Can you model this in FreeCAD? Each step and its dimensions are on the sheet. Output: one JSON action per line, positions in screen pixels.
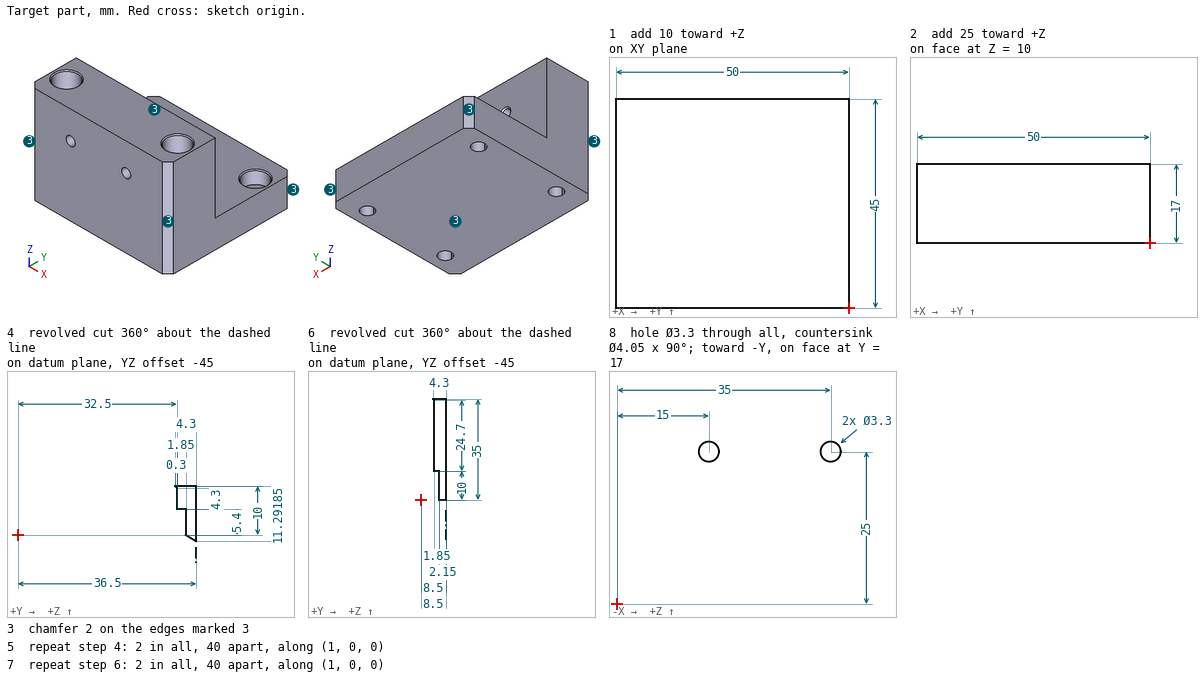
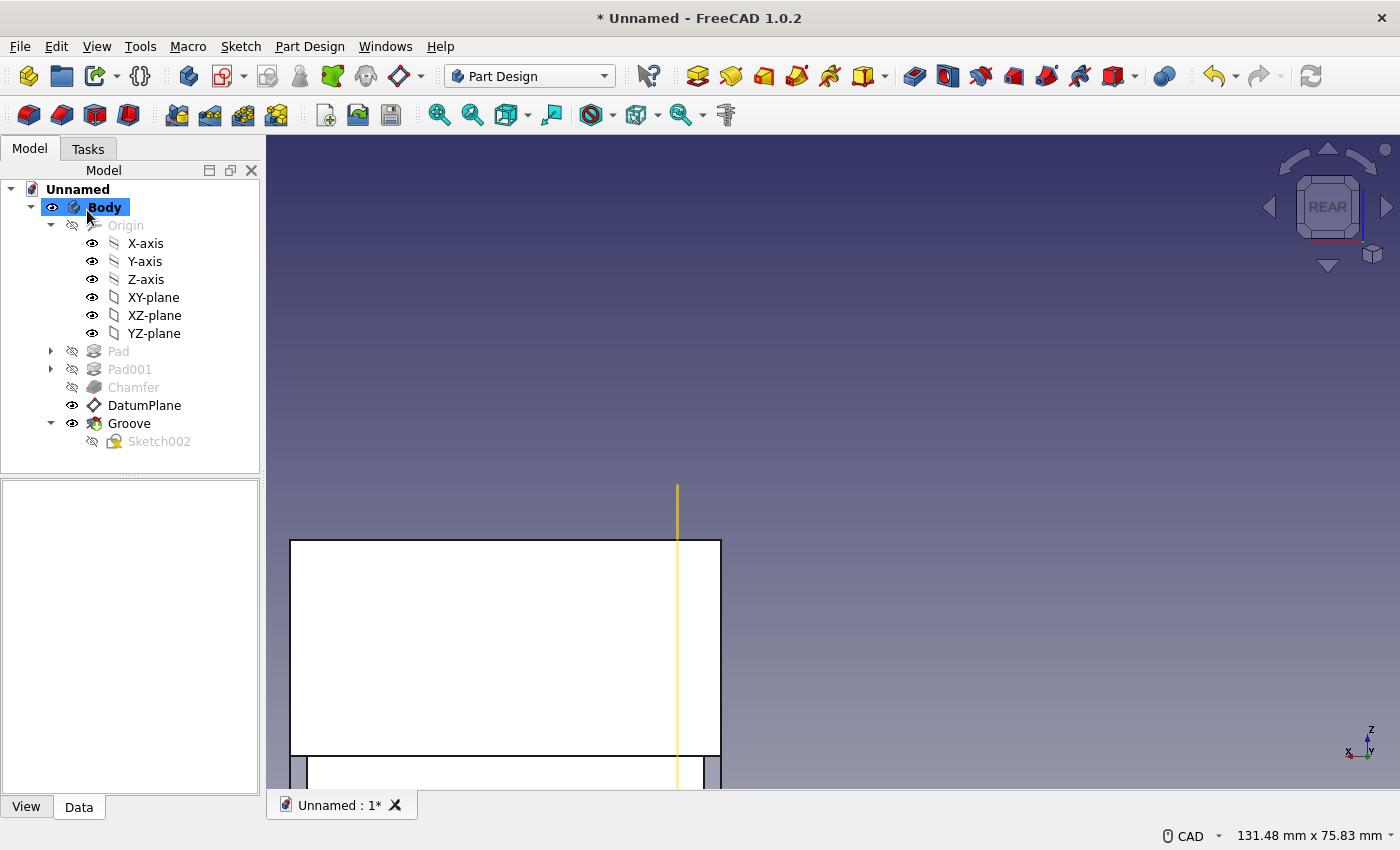
{"action": "left_click", "coordinate": [117, 405]}
{"action": "key", "text": "space"}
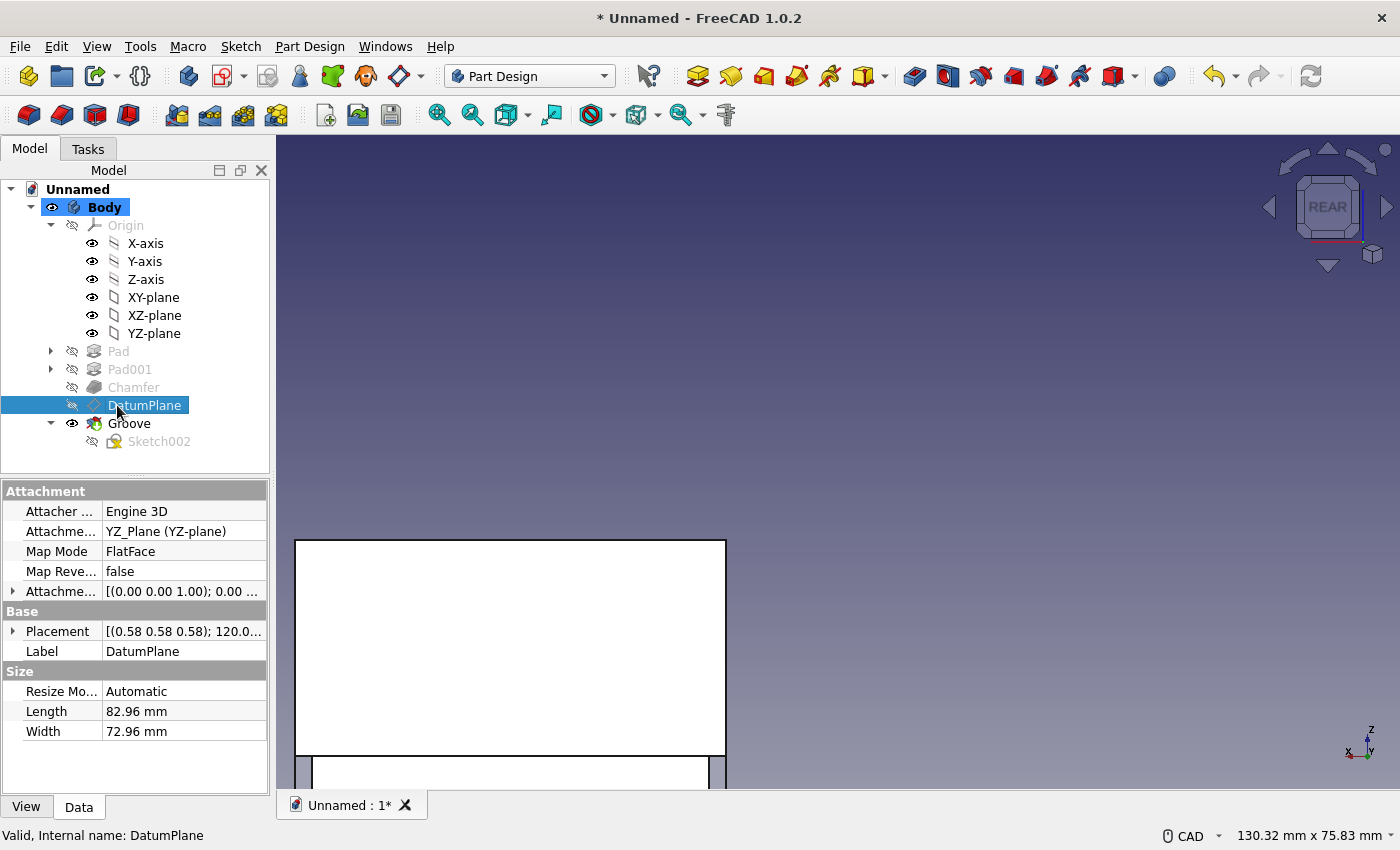
{"action": "key", "text": "v f"}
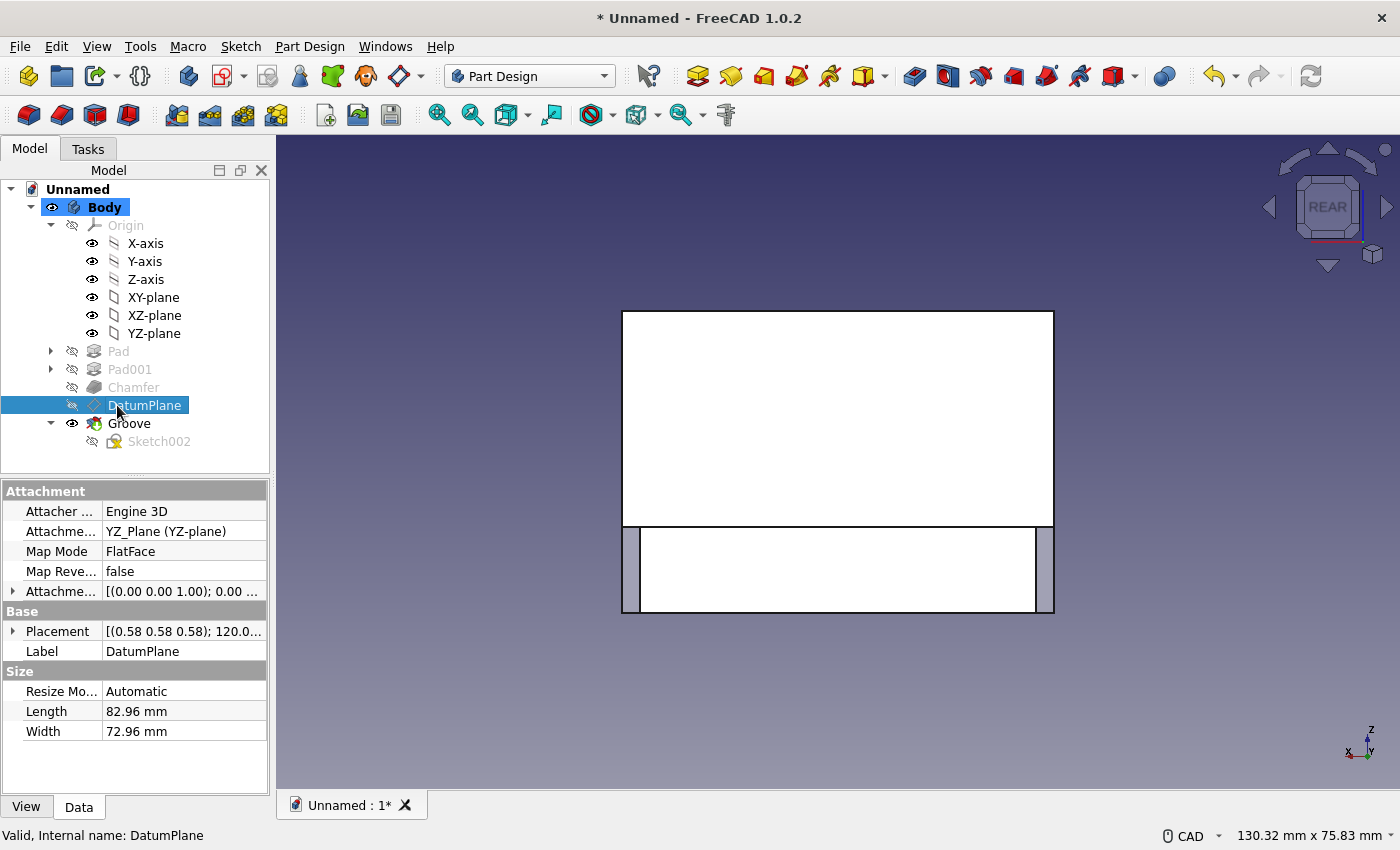
{"action": "left_click", "coordinate": [117, 423]}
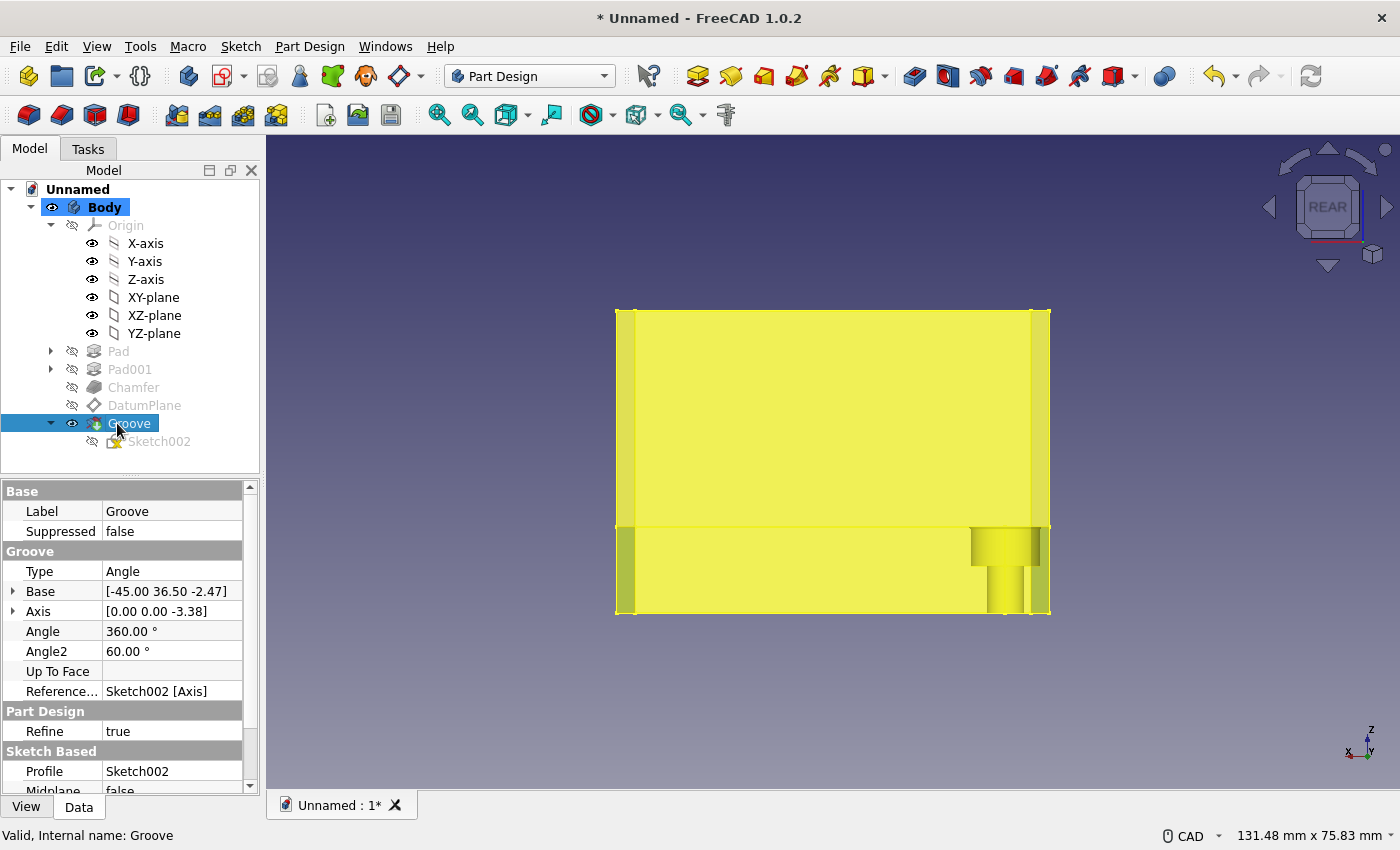
{"action": "left_click", "coordinate": [210, 116]}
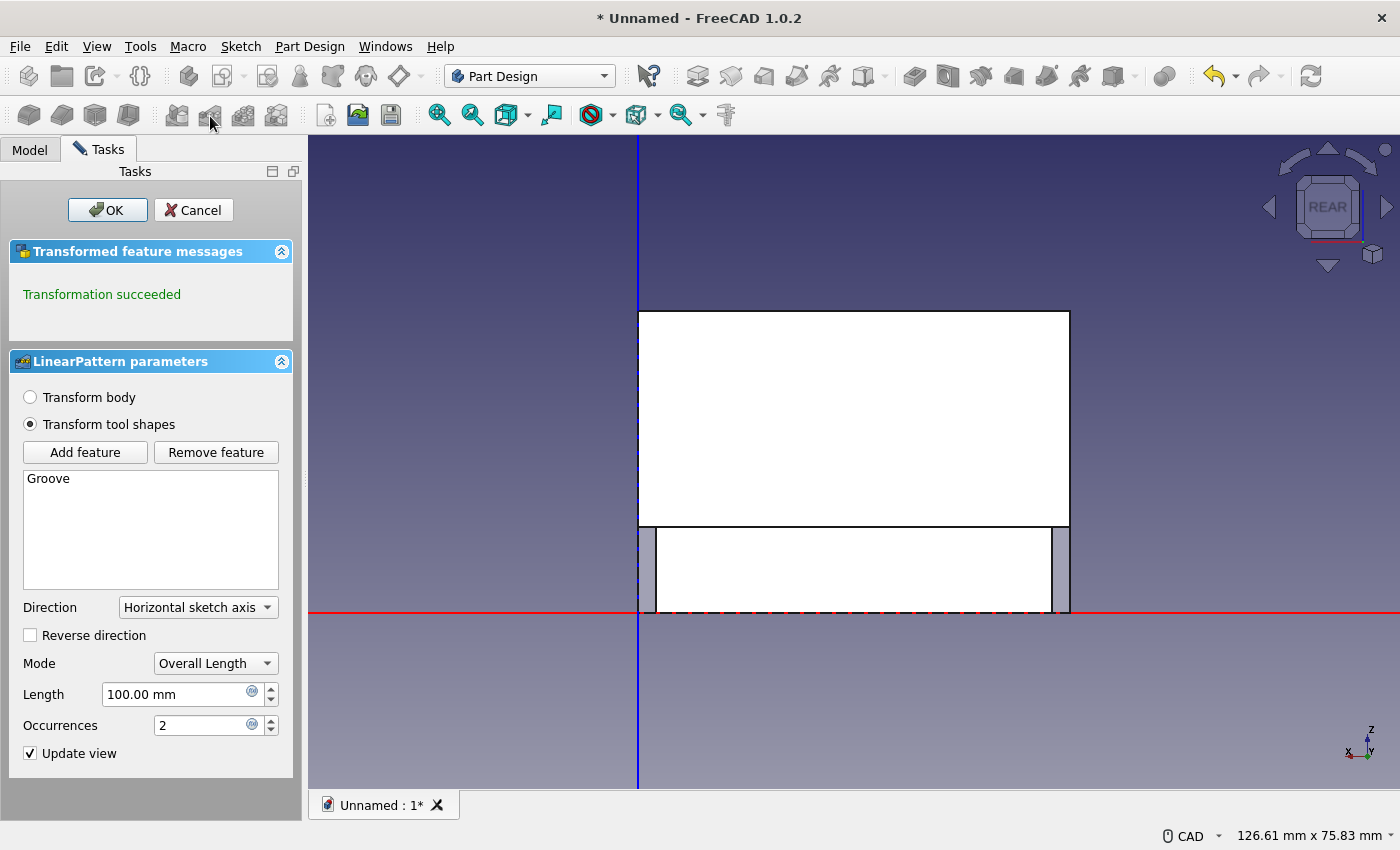
{"action": "left_click", "coordinate": [199, 608]}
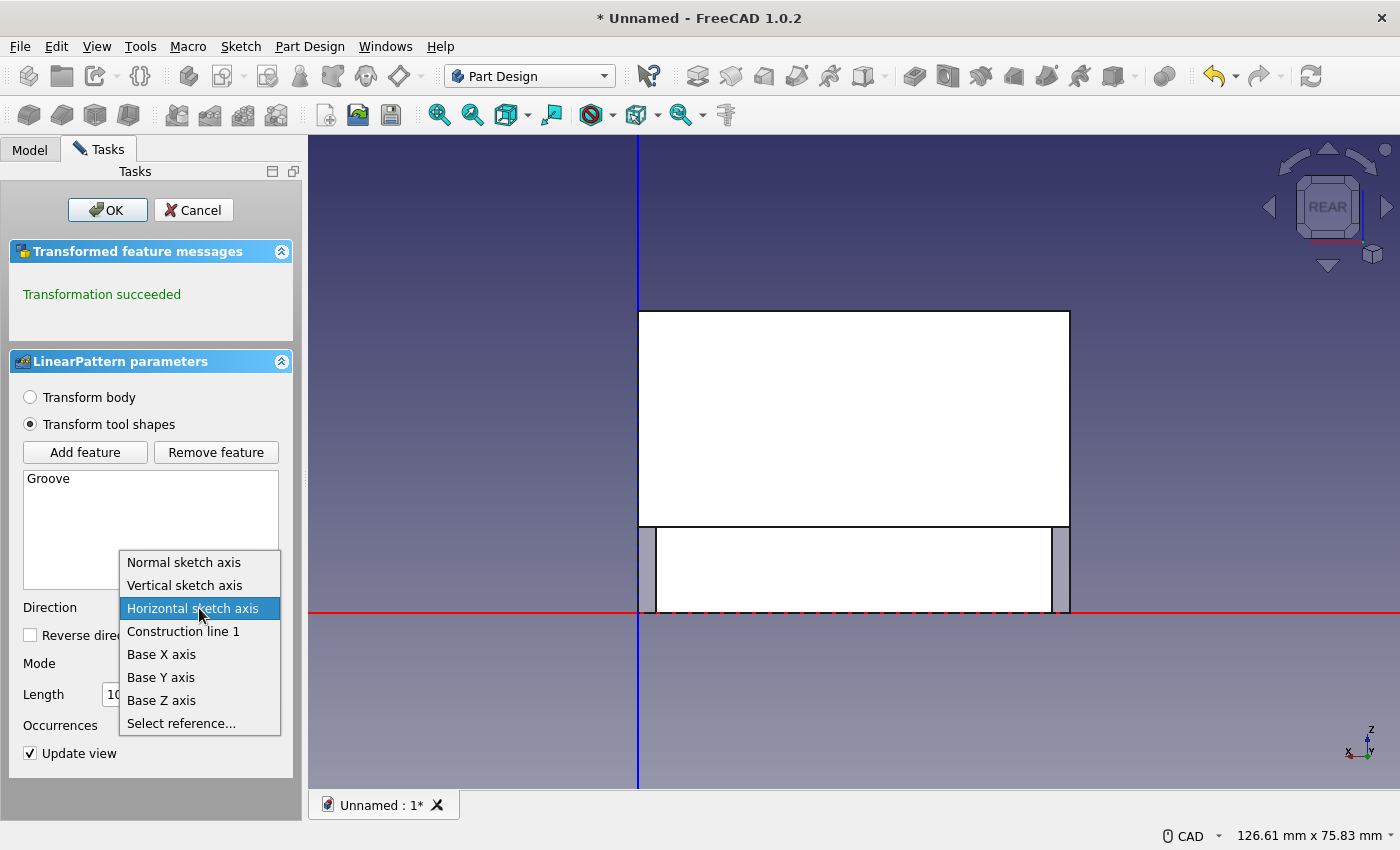
{"action": "left_click", "coordinate": [198, 654]}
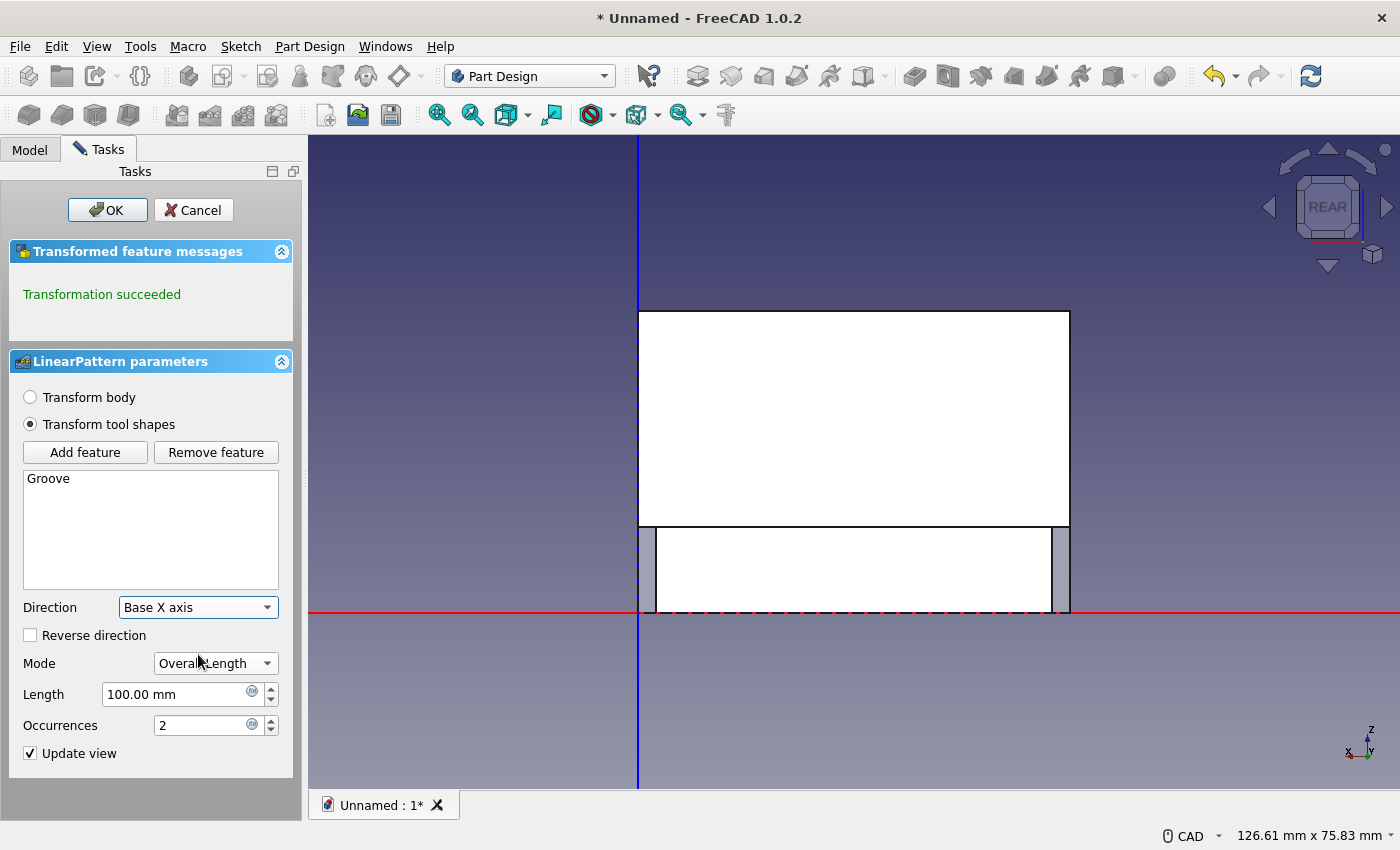
{"action": "left_click", "coordinate": [216, 664]}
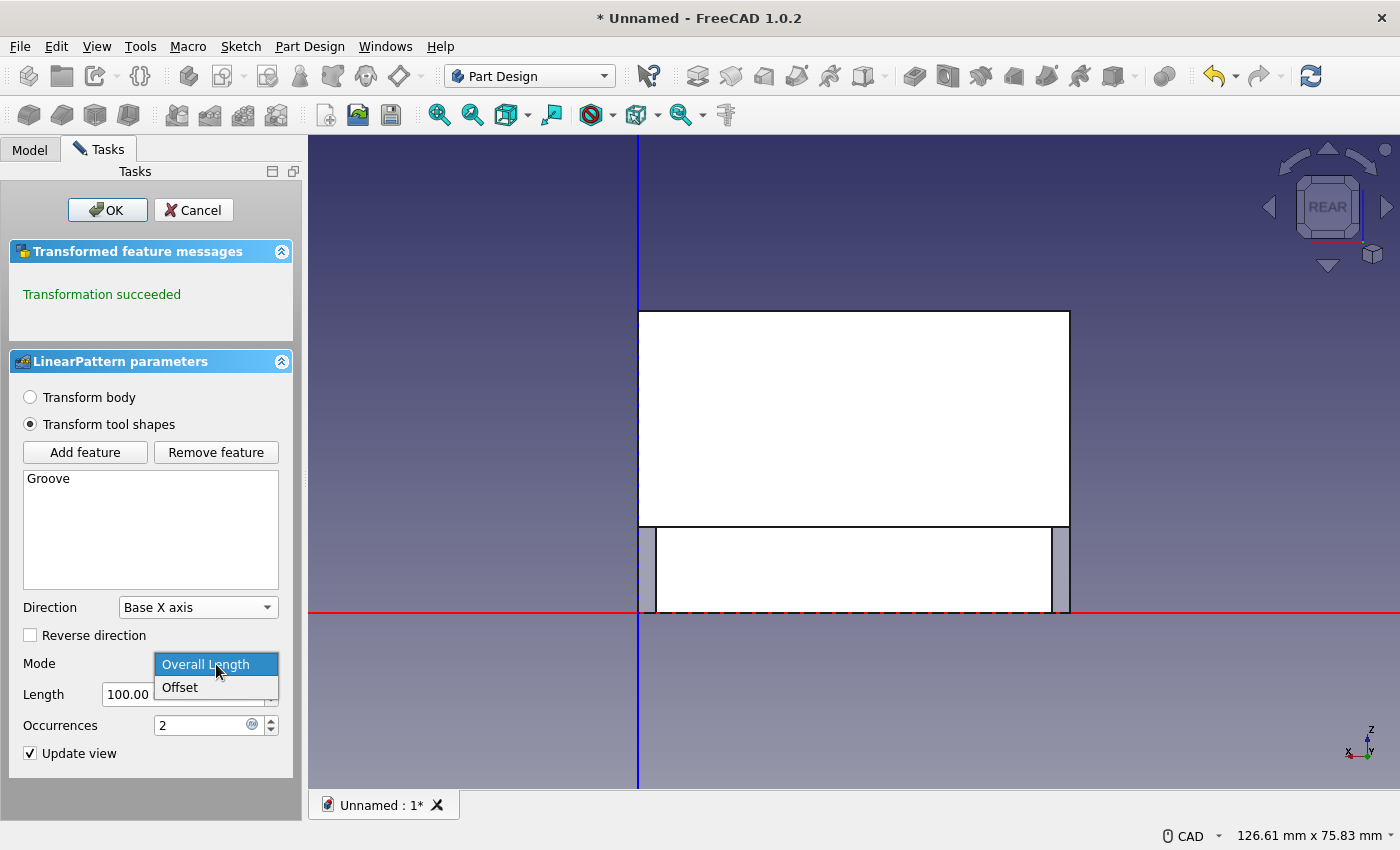
{"action": "left_click", "coordinate": [214, 688]}